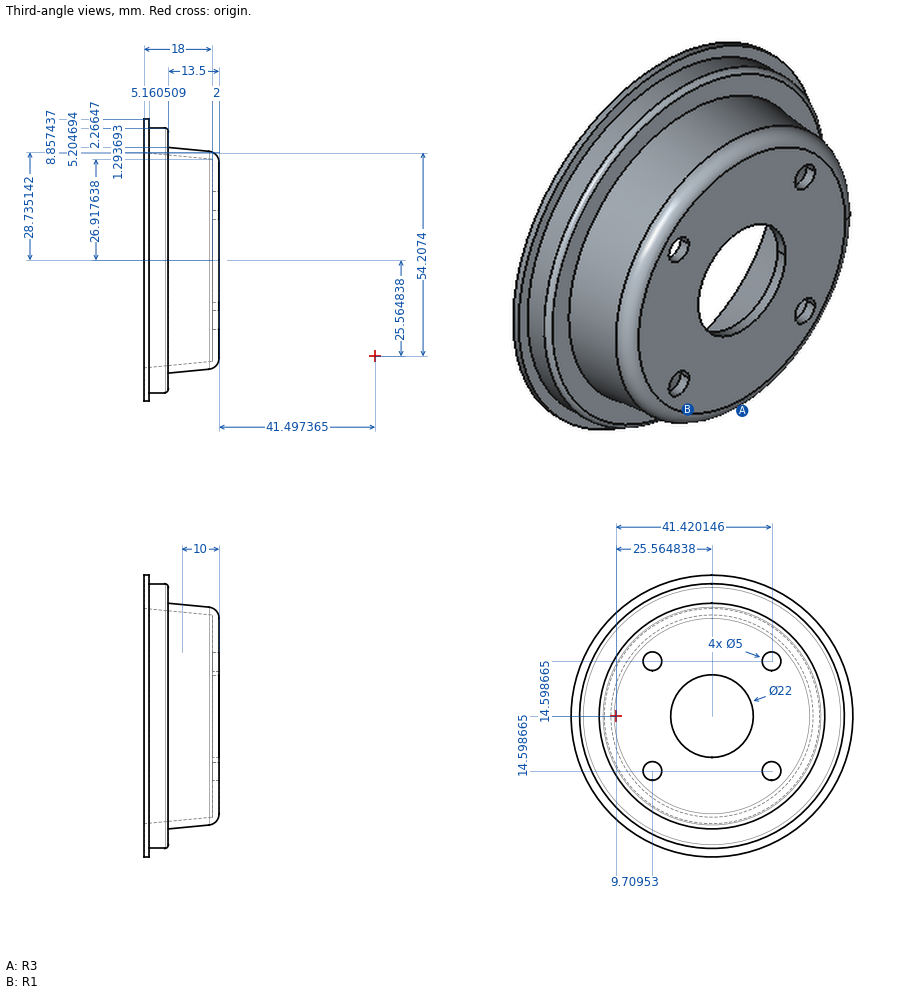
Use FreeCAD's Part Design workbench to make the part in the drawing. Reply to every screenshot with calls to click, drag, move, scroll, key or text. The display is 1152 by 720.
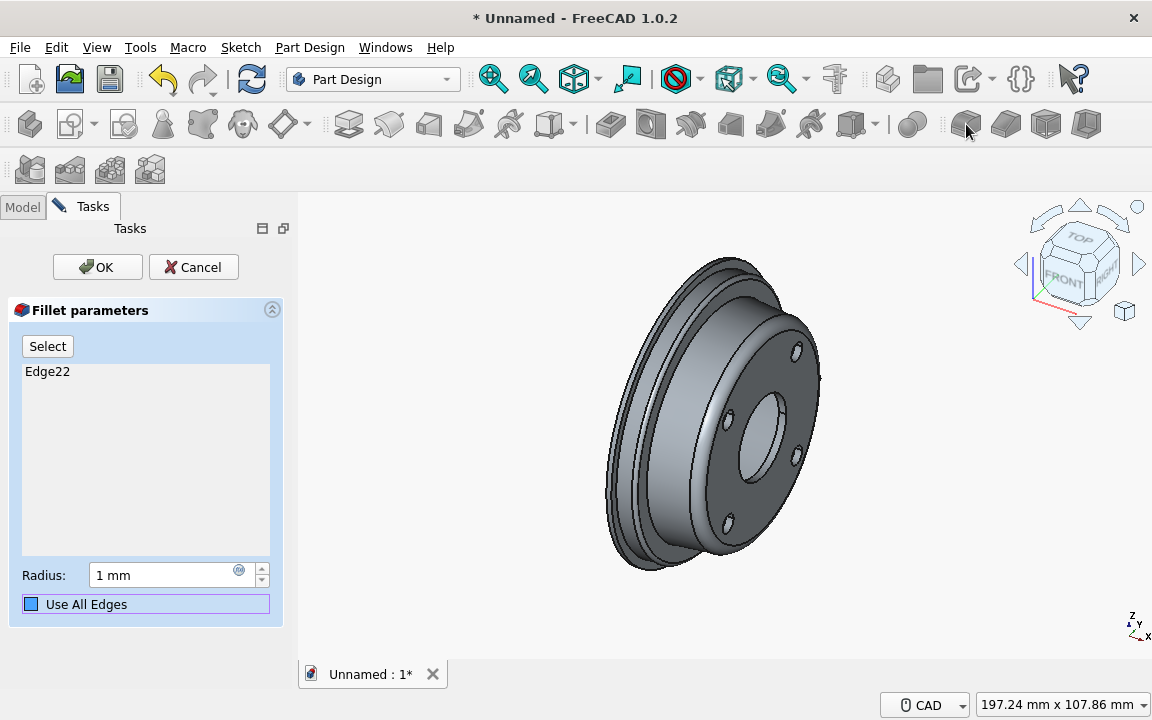
click(98, 267)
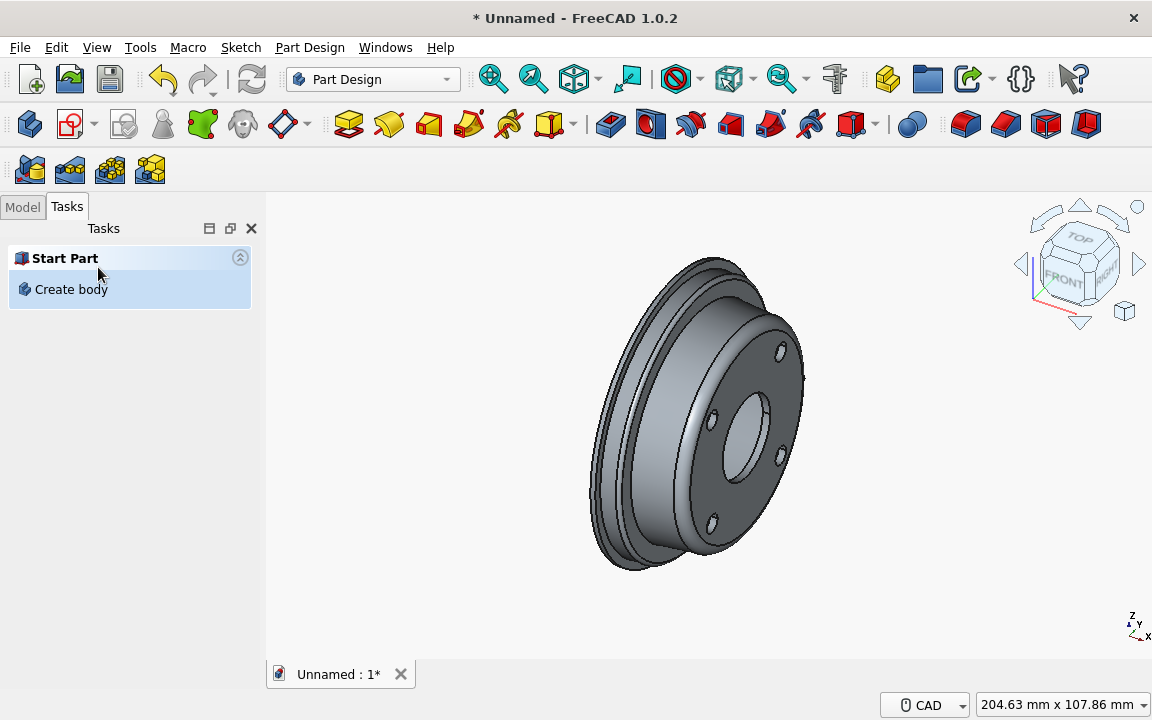
key(0)